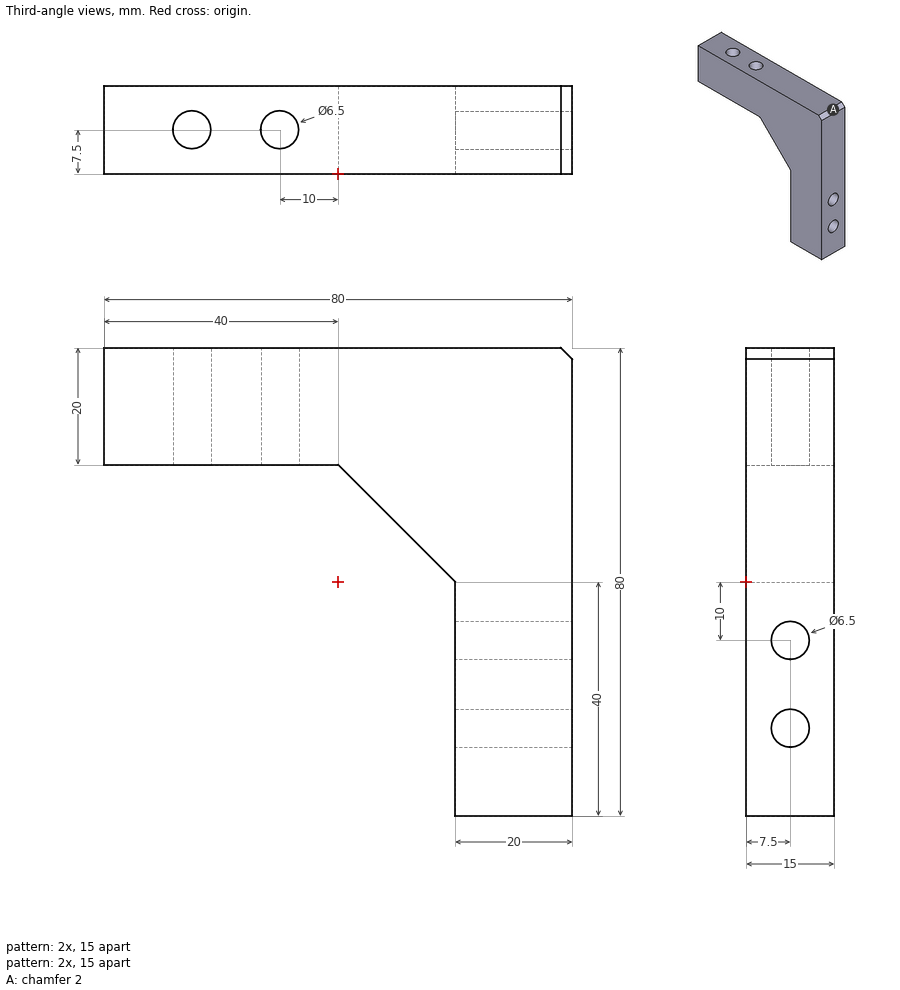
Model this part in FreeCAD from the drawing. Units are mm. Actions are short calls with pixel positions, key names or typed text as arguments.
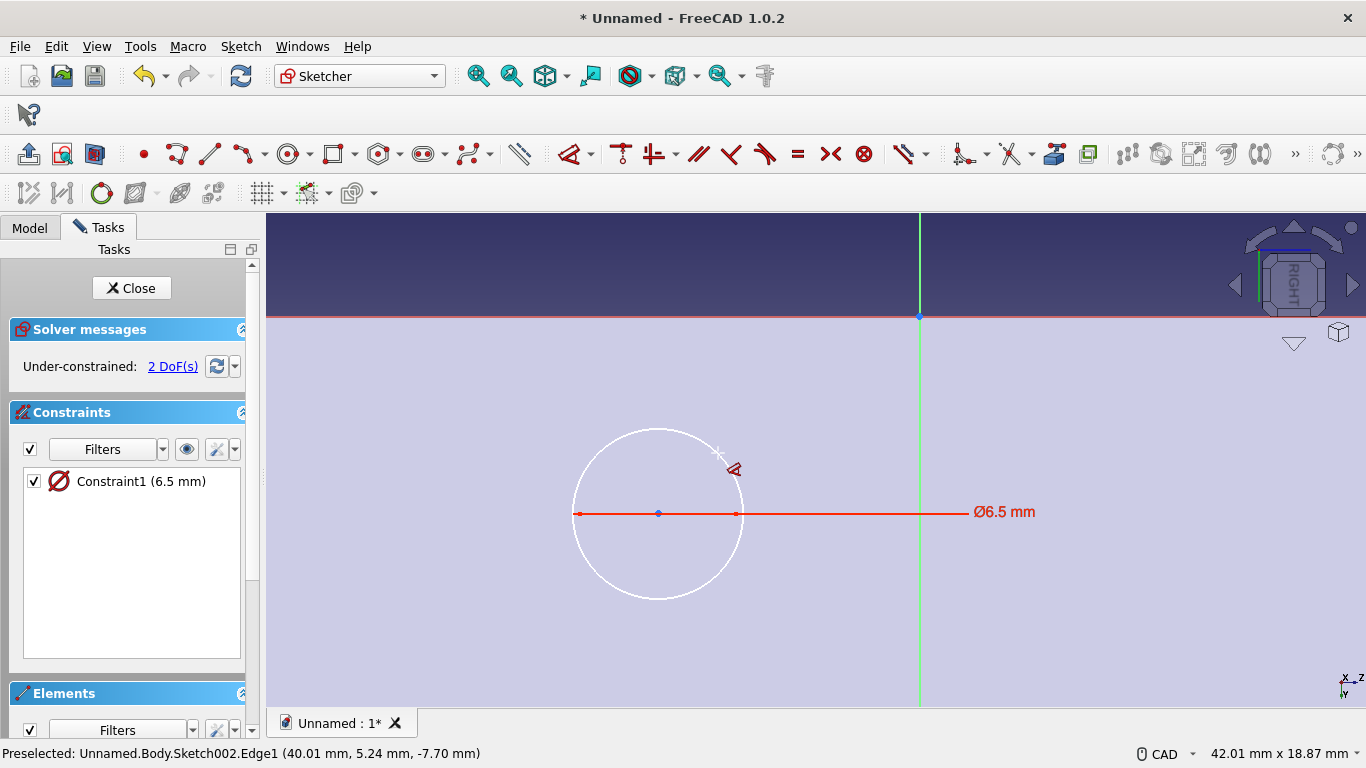
click(658, 514)
click(789, 283)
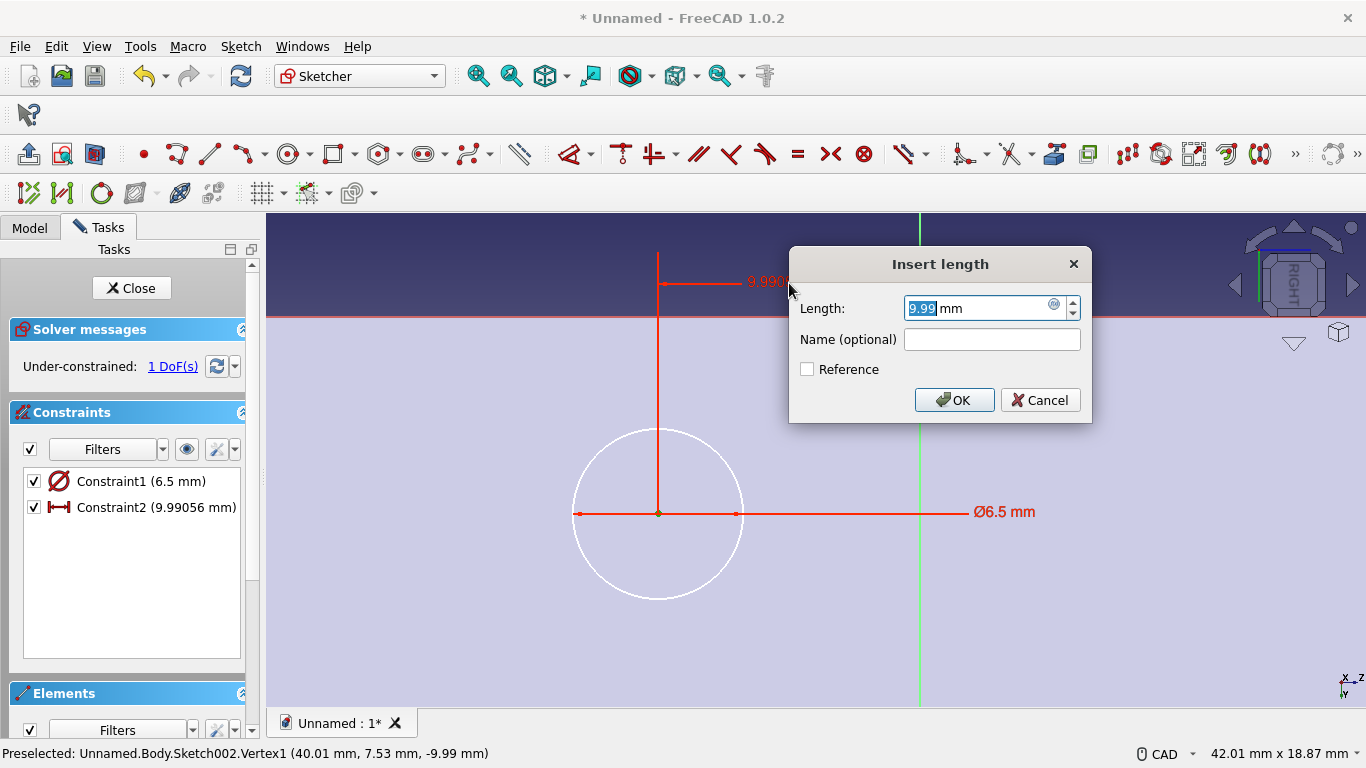
text(10)
key(Return)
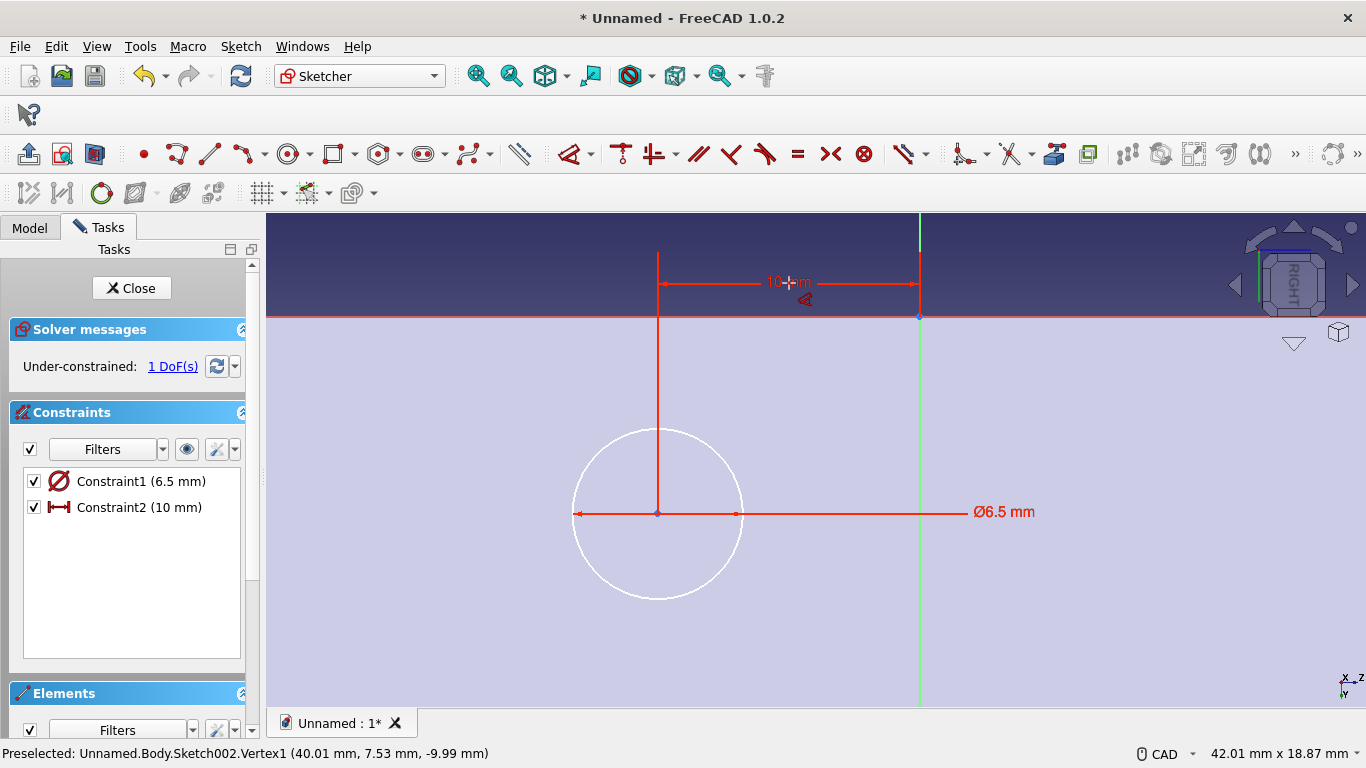
click(658, 514)
click(954, 415)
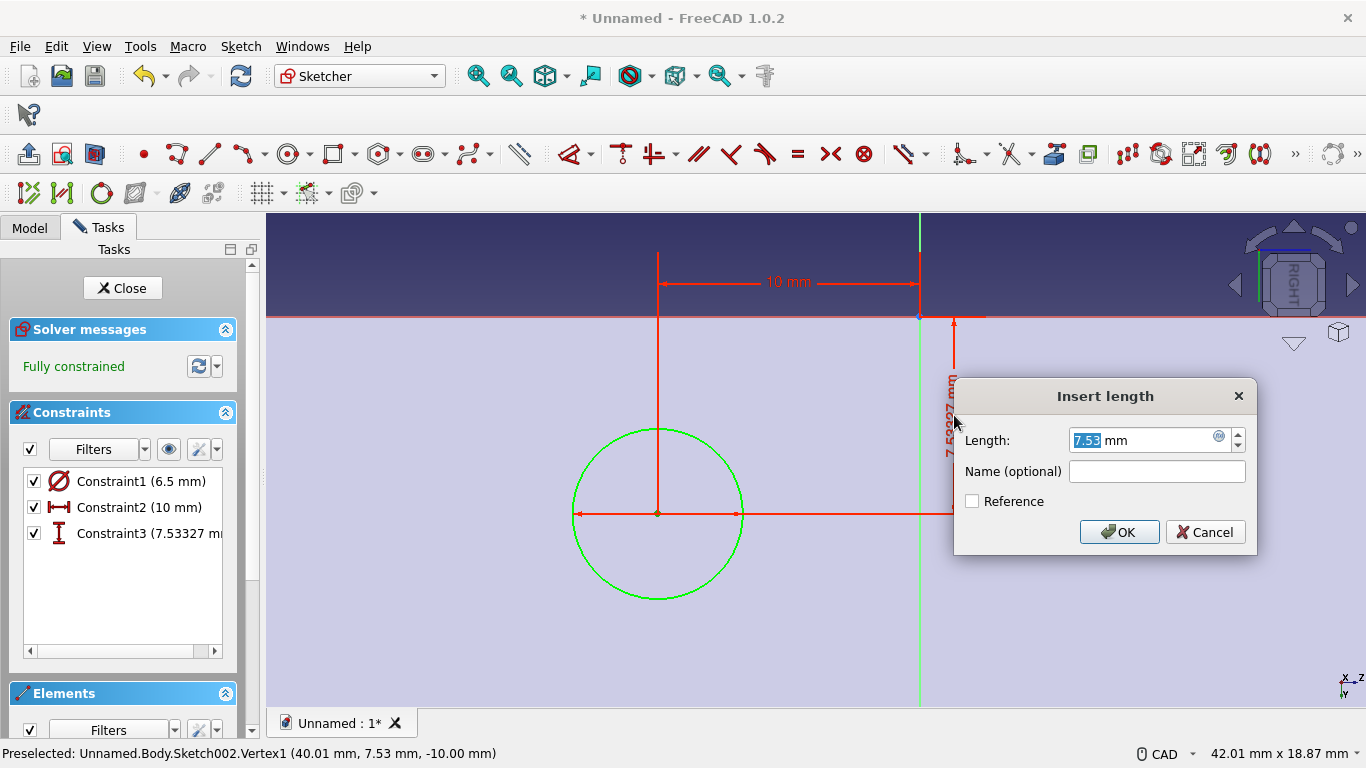
text(7.5)
key(Return)
key(Escape)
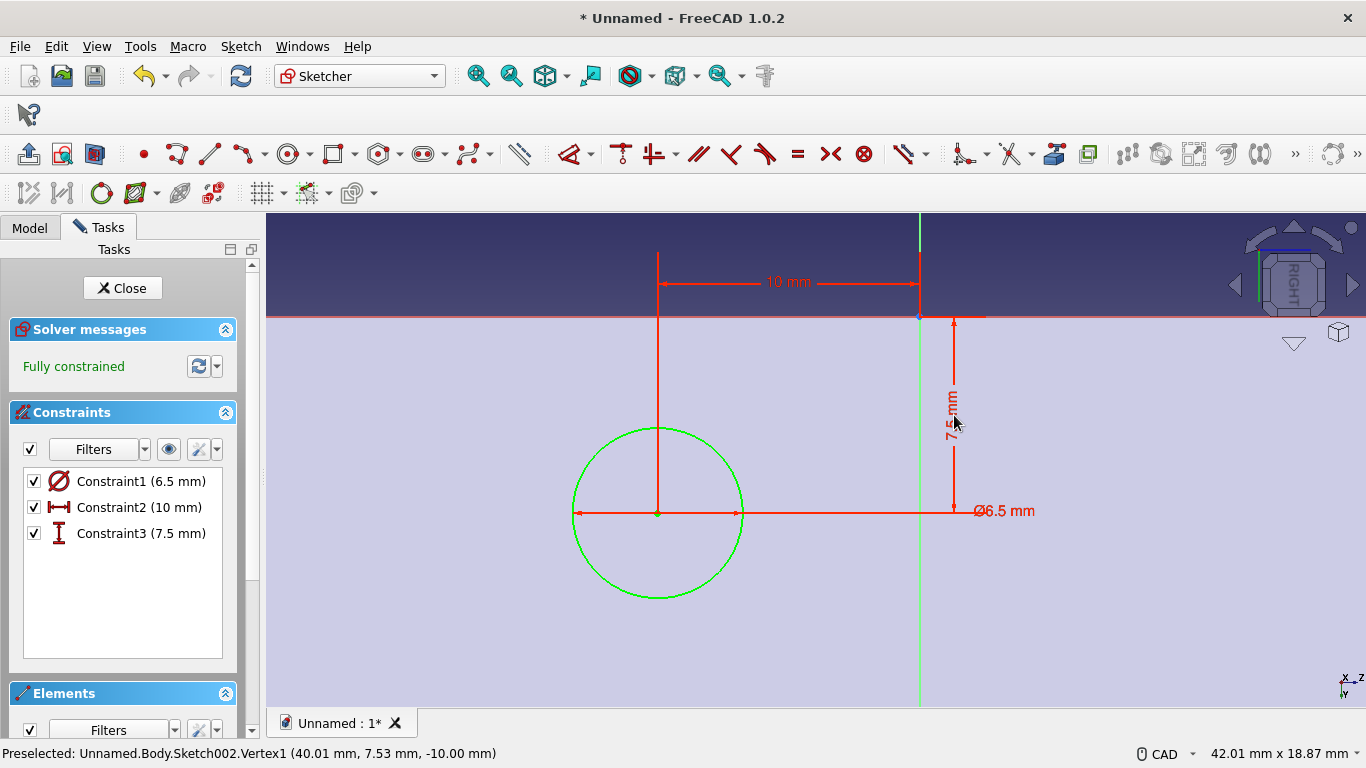
click(123, 288)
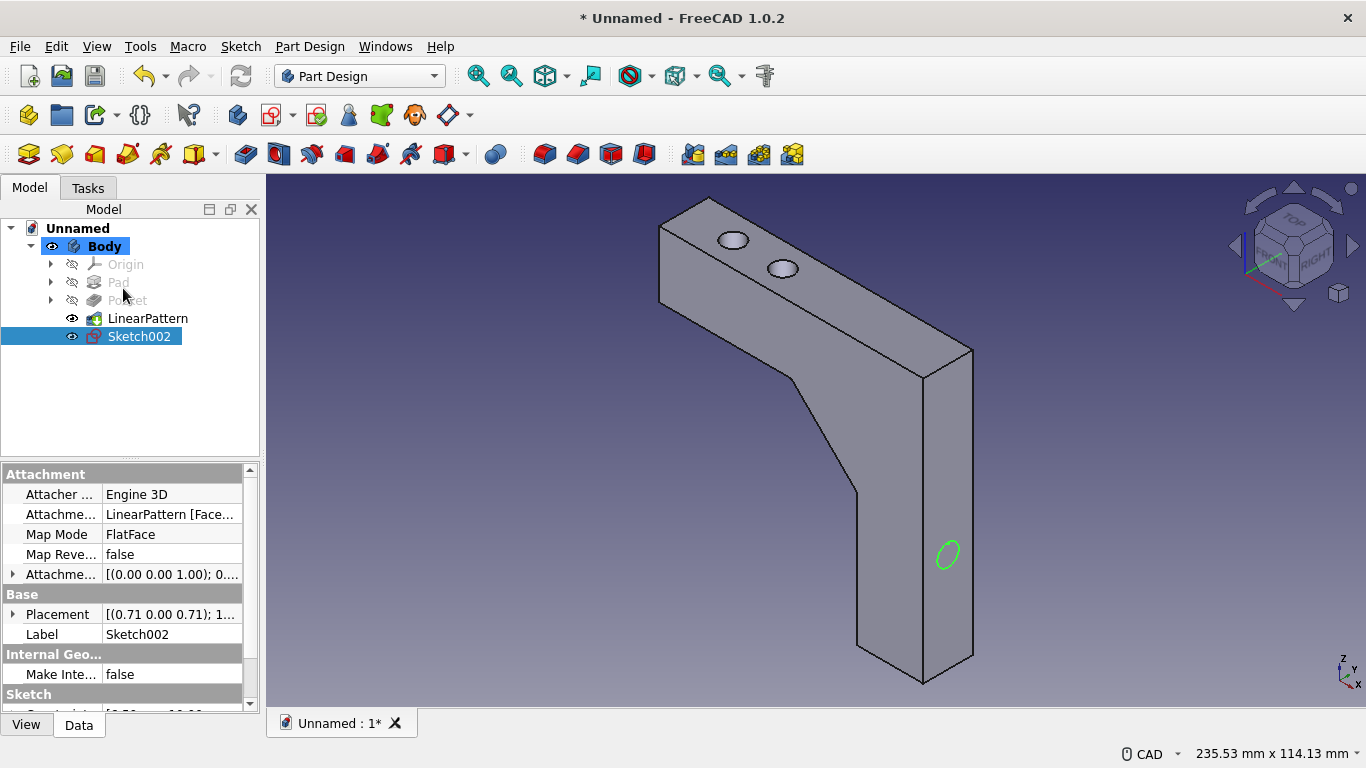
click(246, 154)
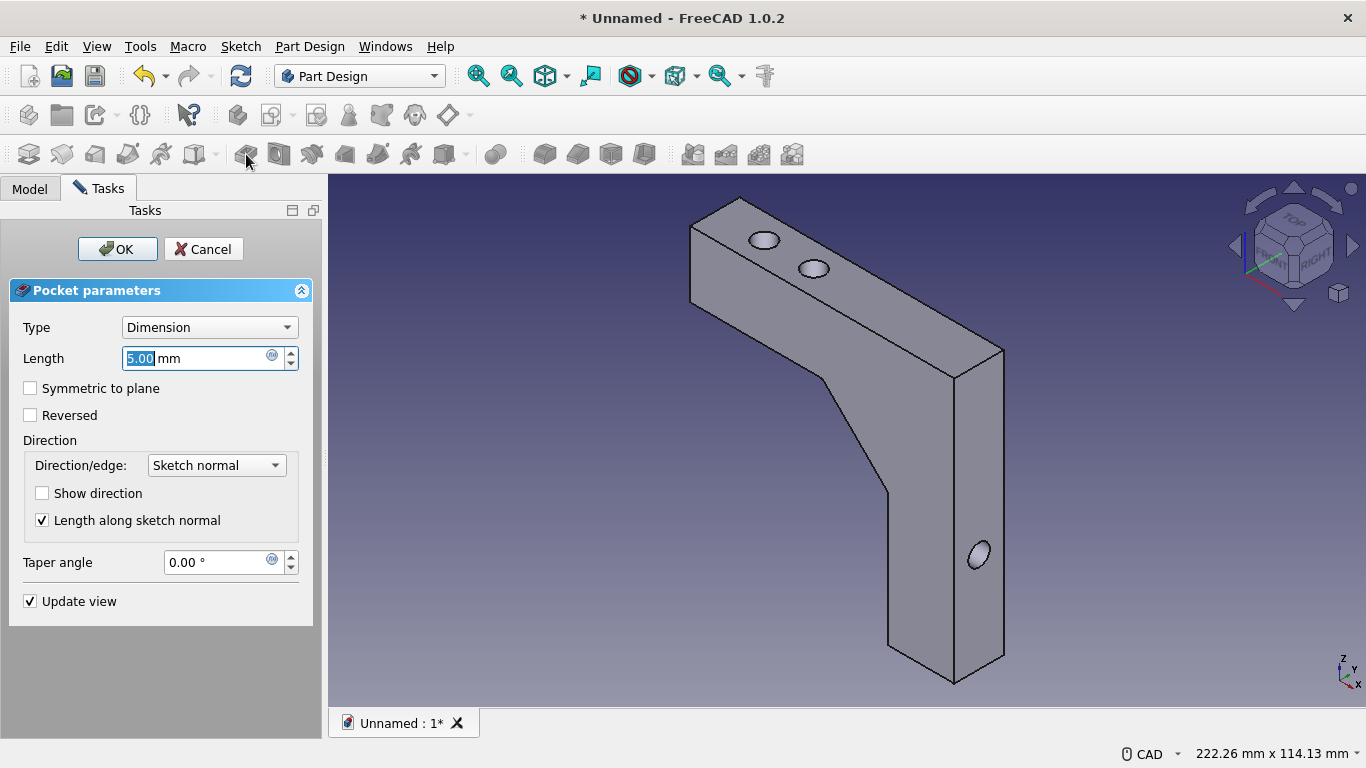
click(210, 328)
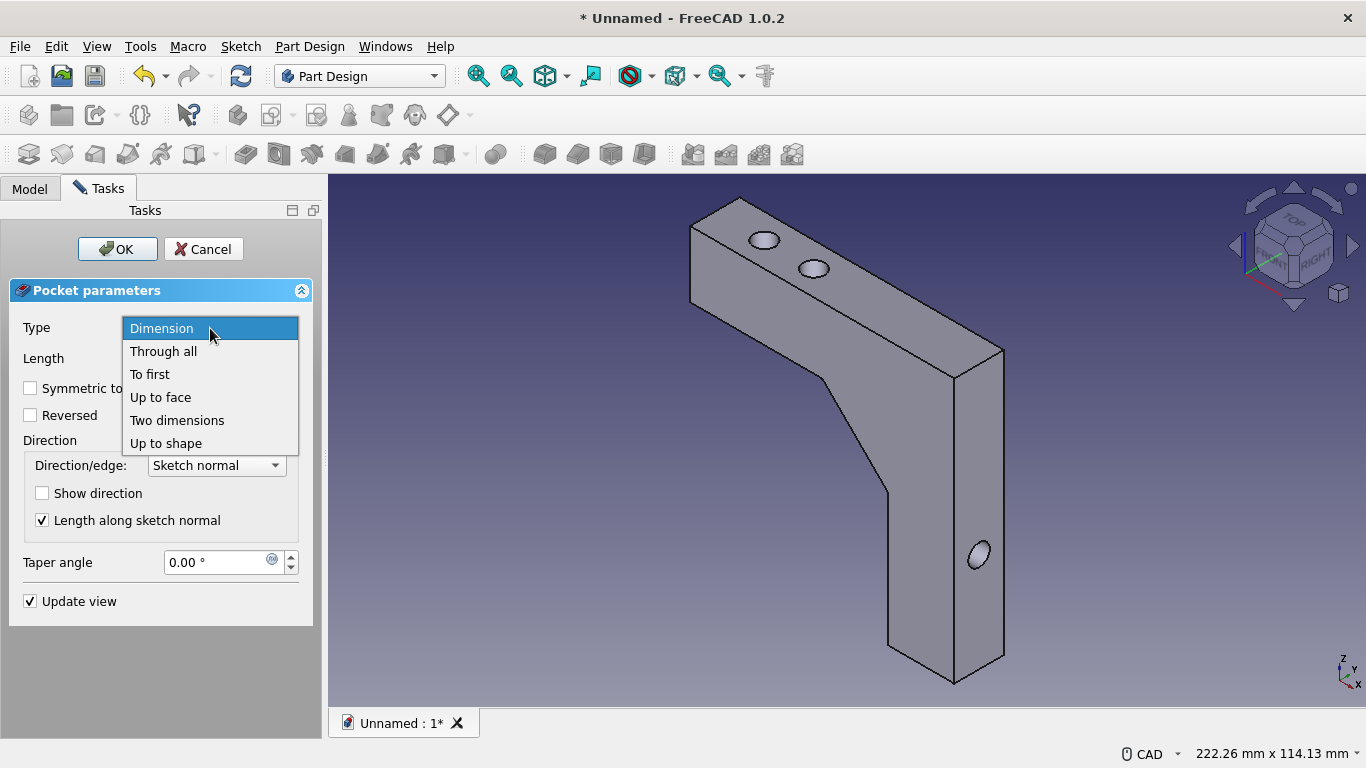
click(208, 352)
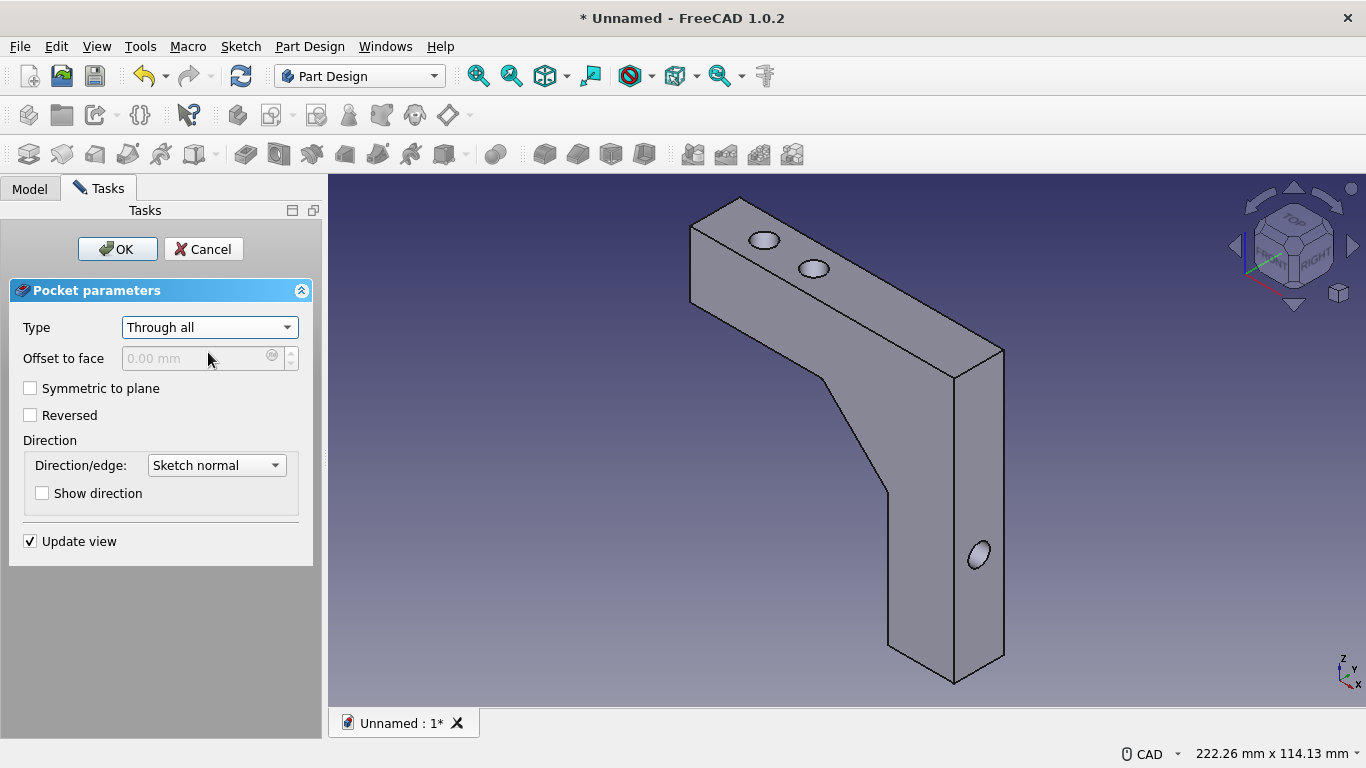
click(118, 249)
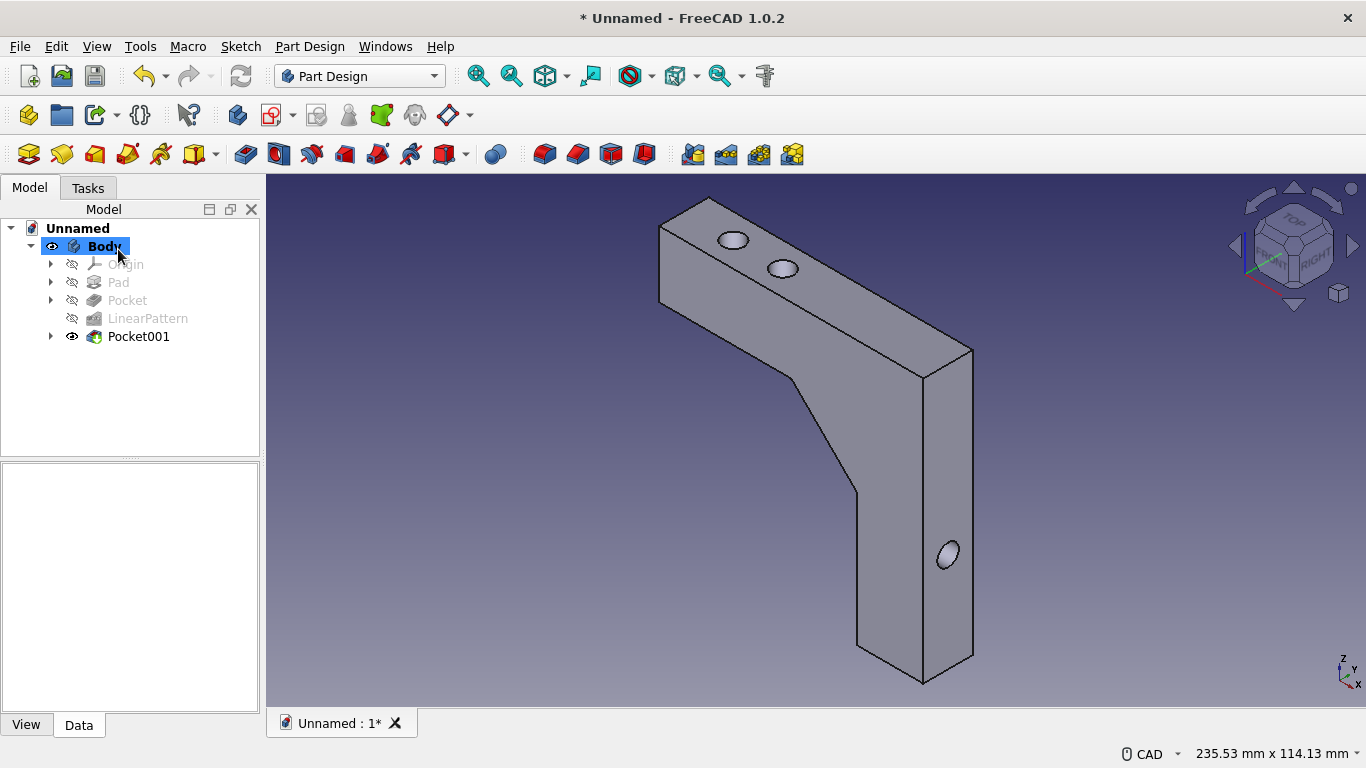
click(117, 336)